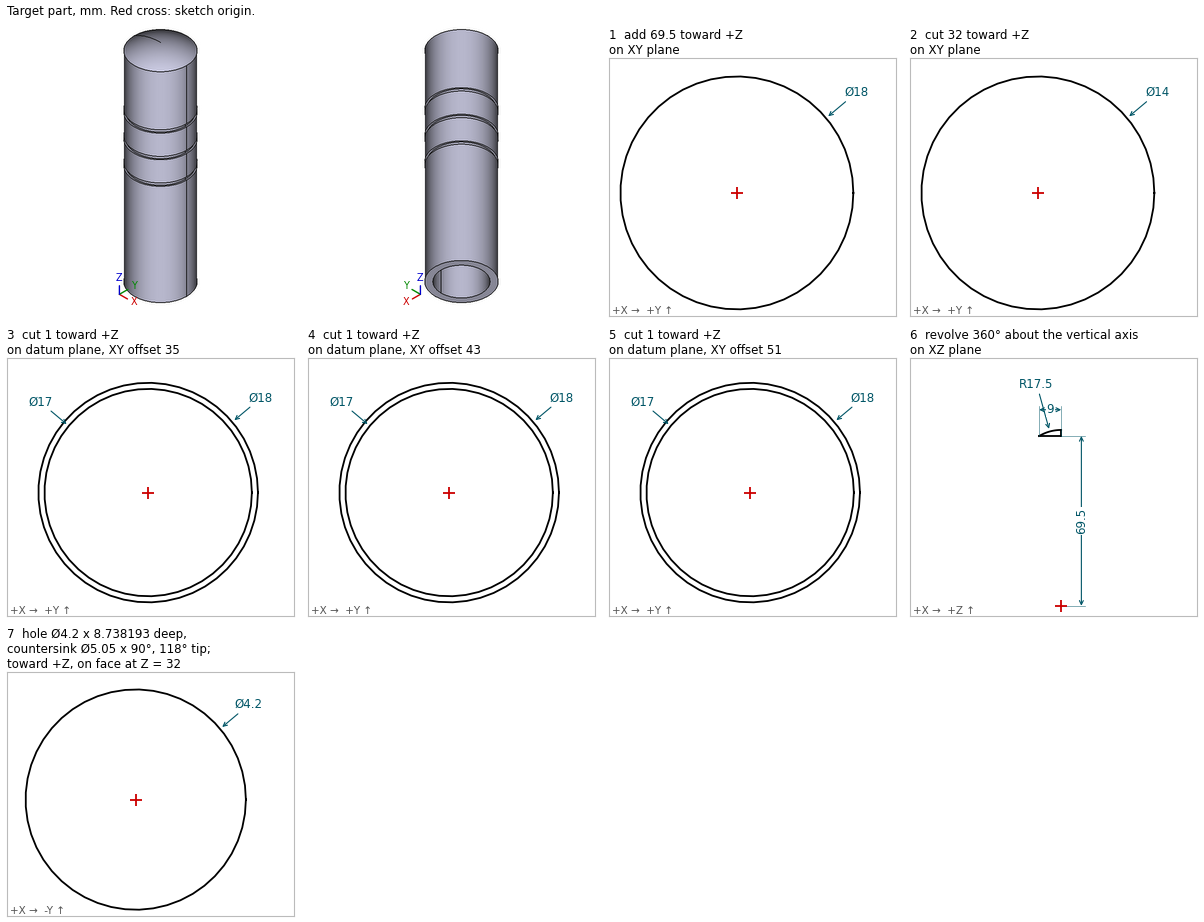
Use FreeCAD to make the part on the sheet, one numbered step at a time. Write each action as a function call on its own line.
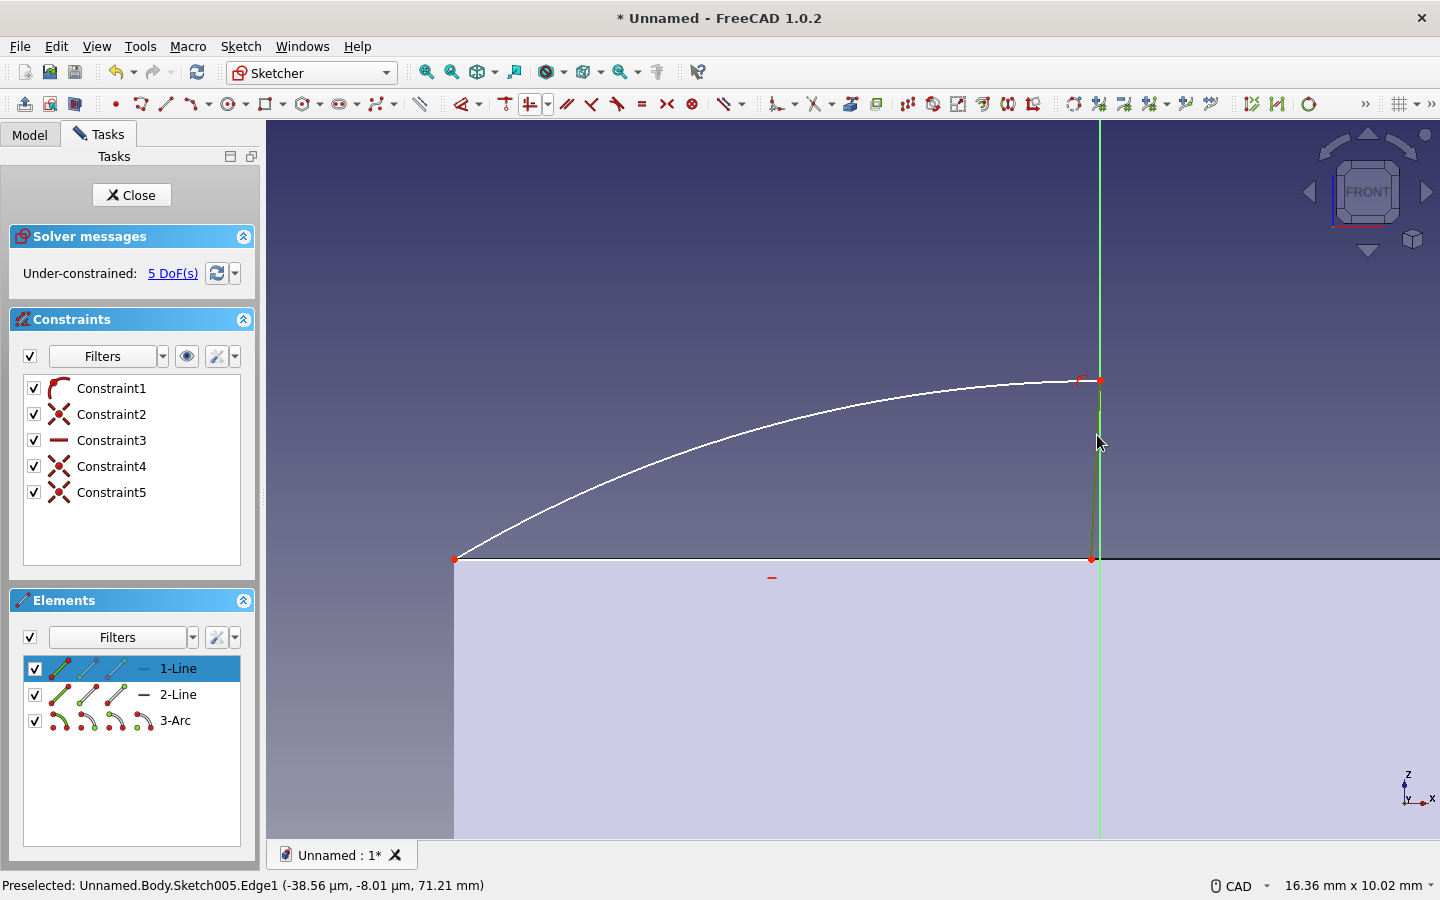
key(v)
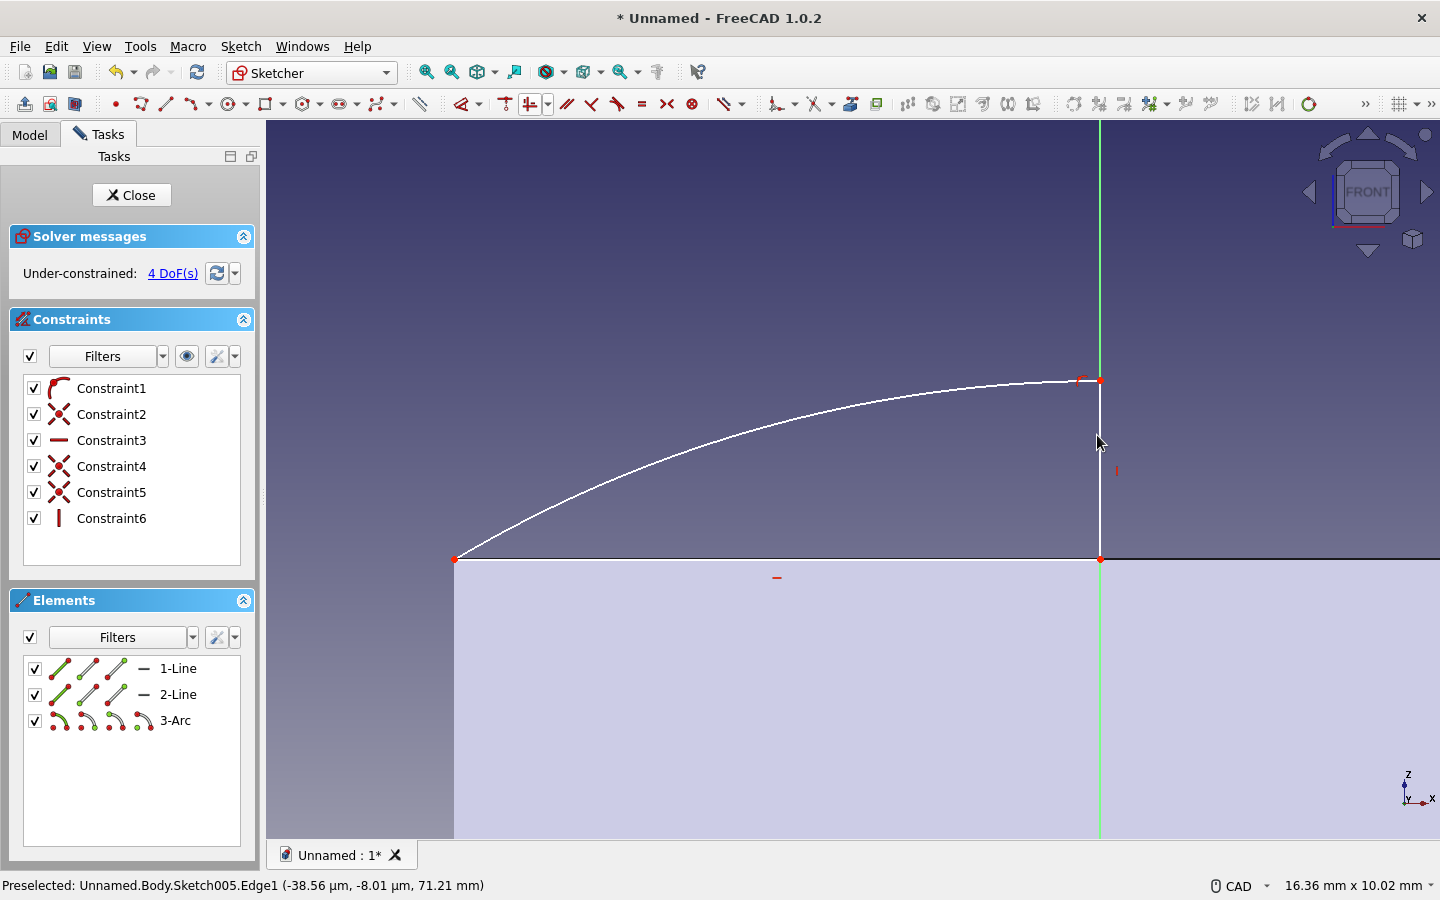
scroll(788, 168, down, 5)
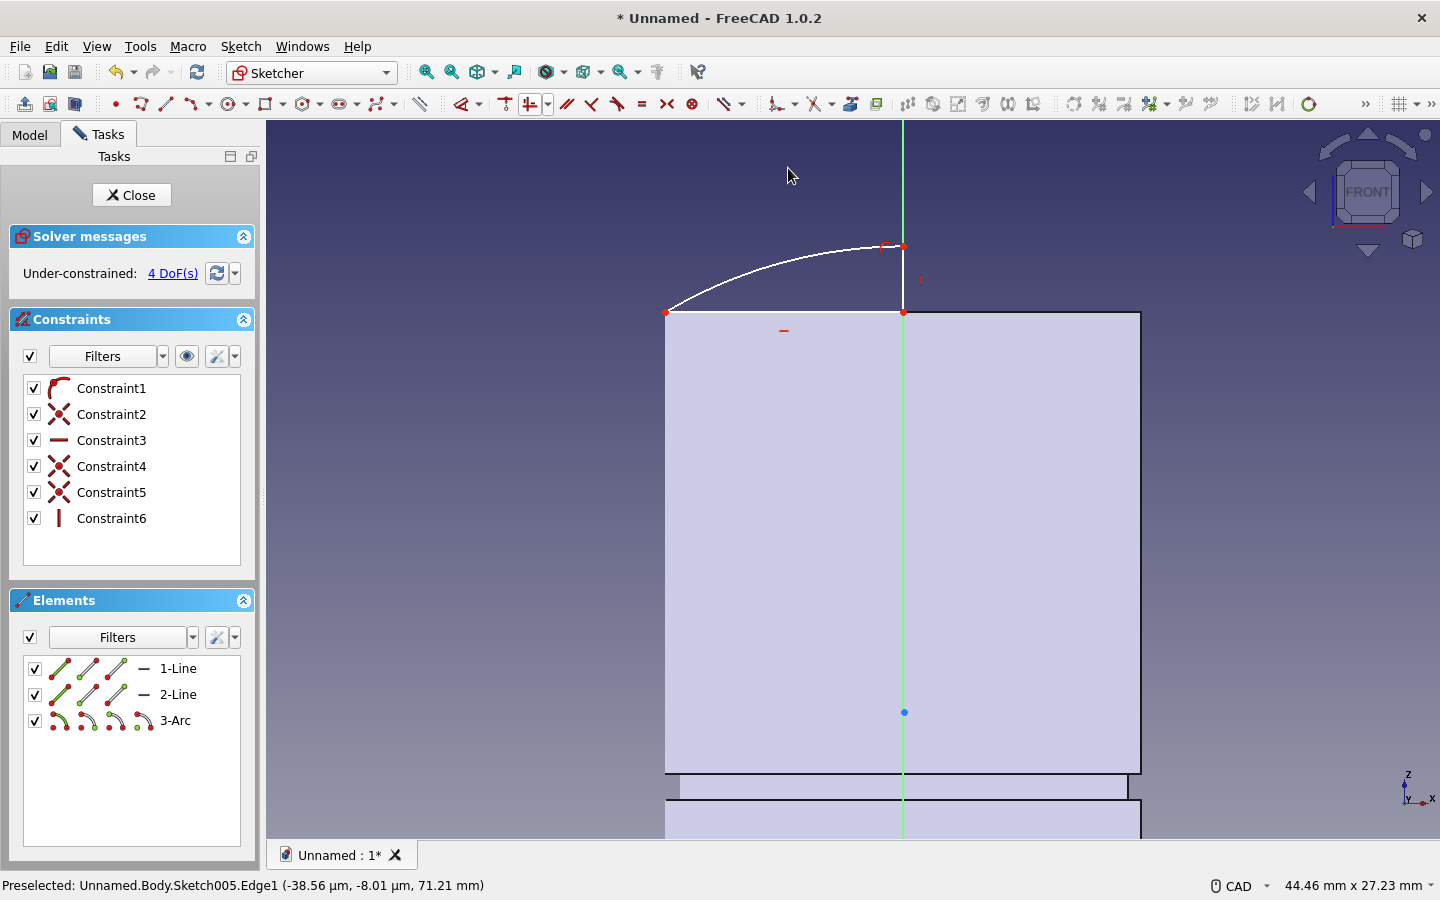
click(904, 713)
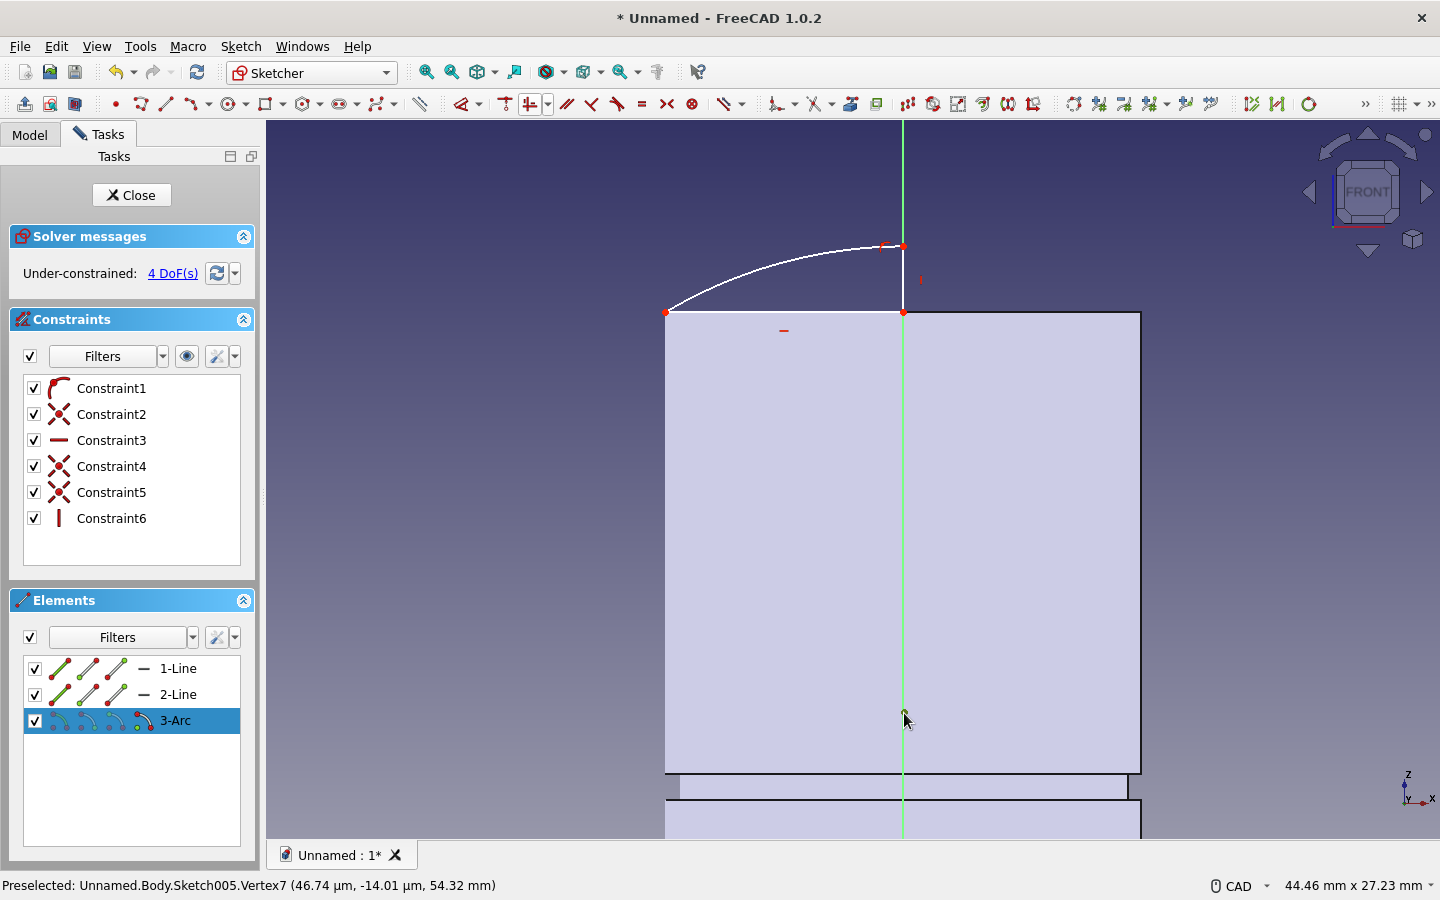
click(903, 764)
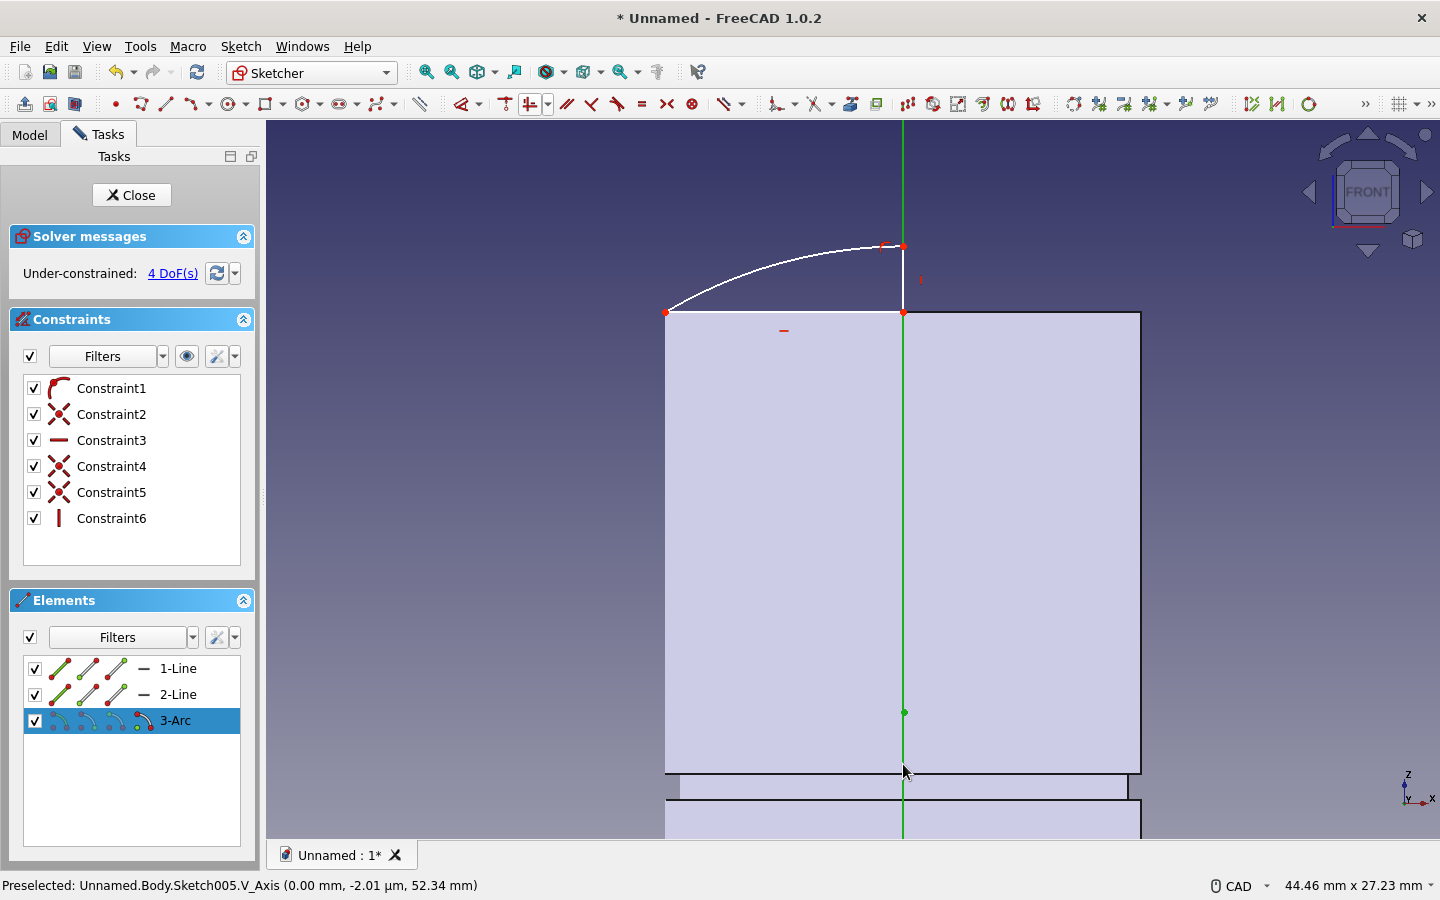
key(c)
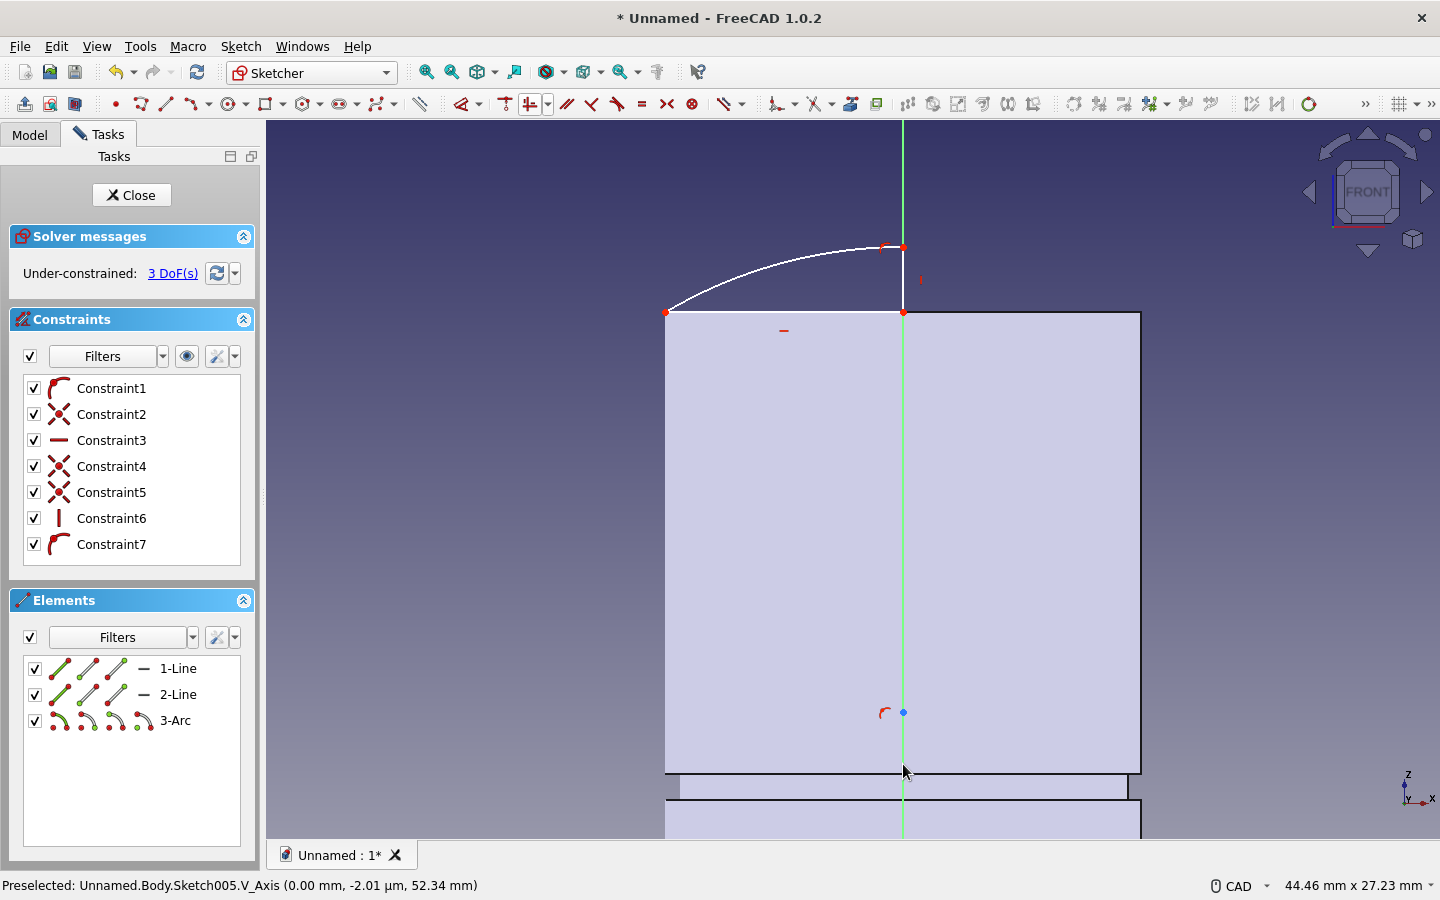
key(d)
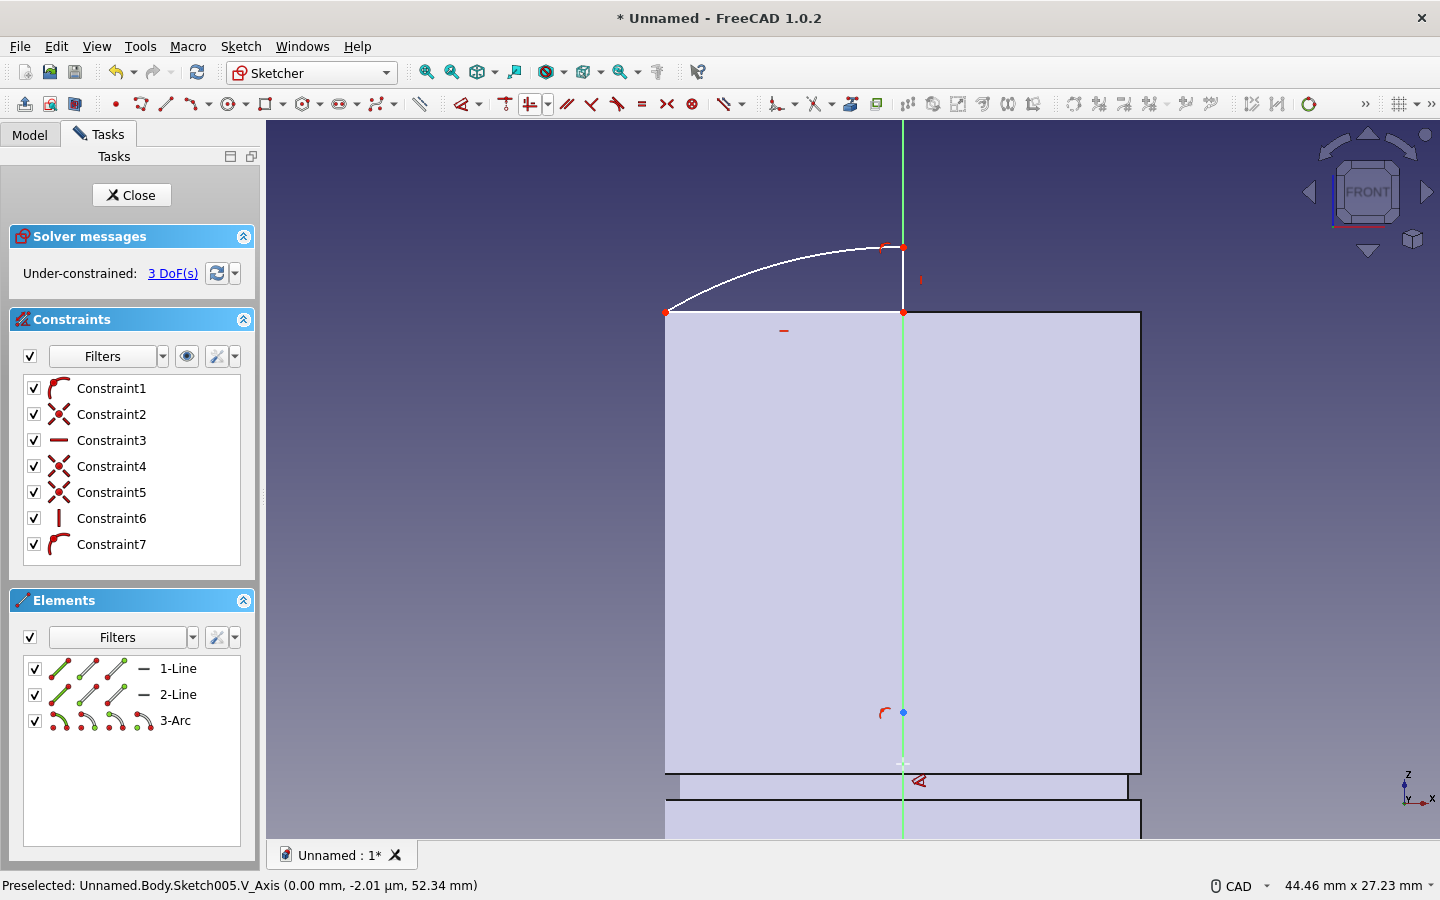
click(829, 253)
click(824, 221)